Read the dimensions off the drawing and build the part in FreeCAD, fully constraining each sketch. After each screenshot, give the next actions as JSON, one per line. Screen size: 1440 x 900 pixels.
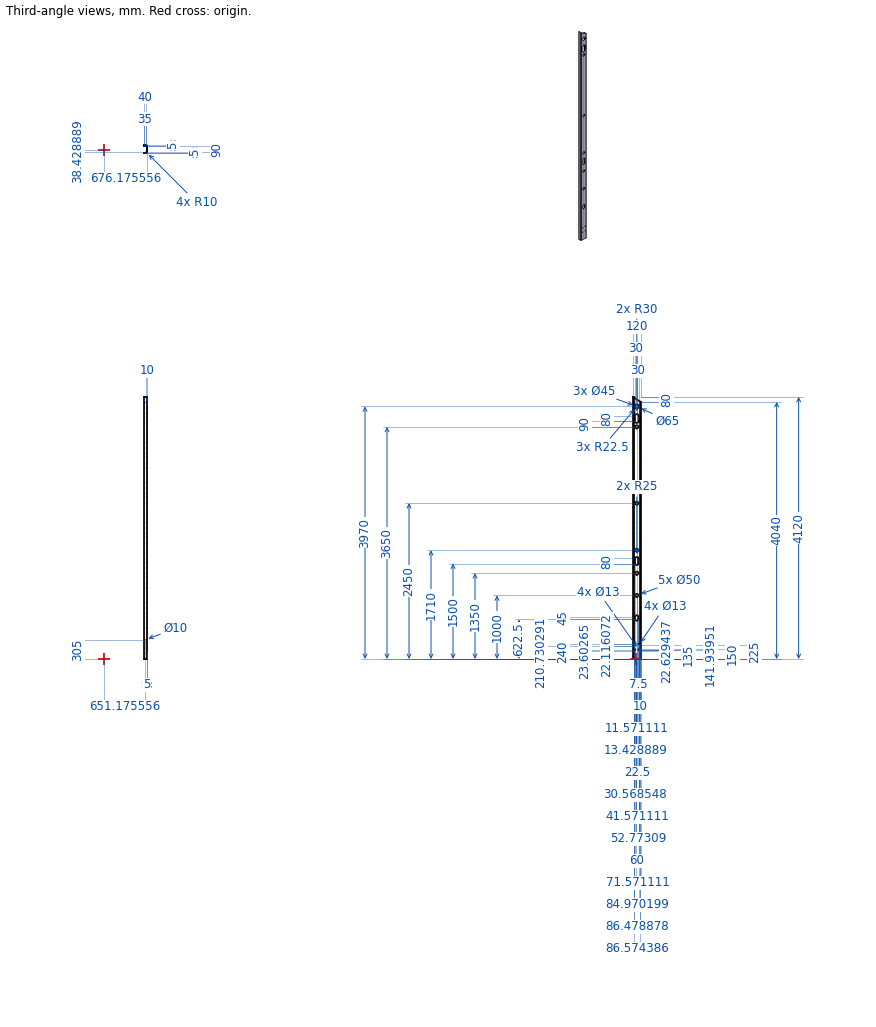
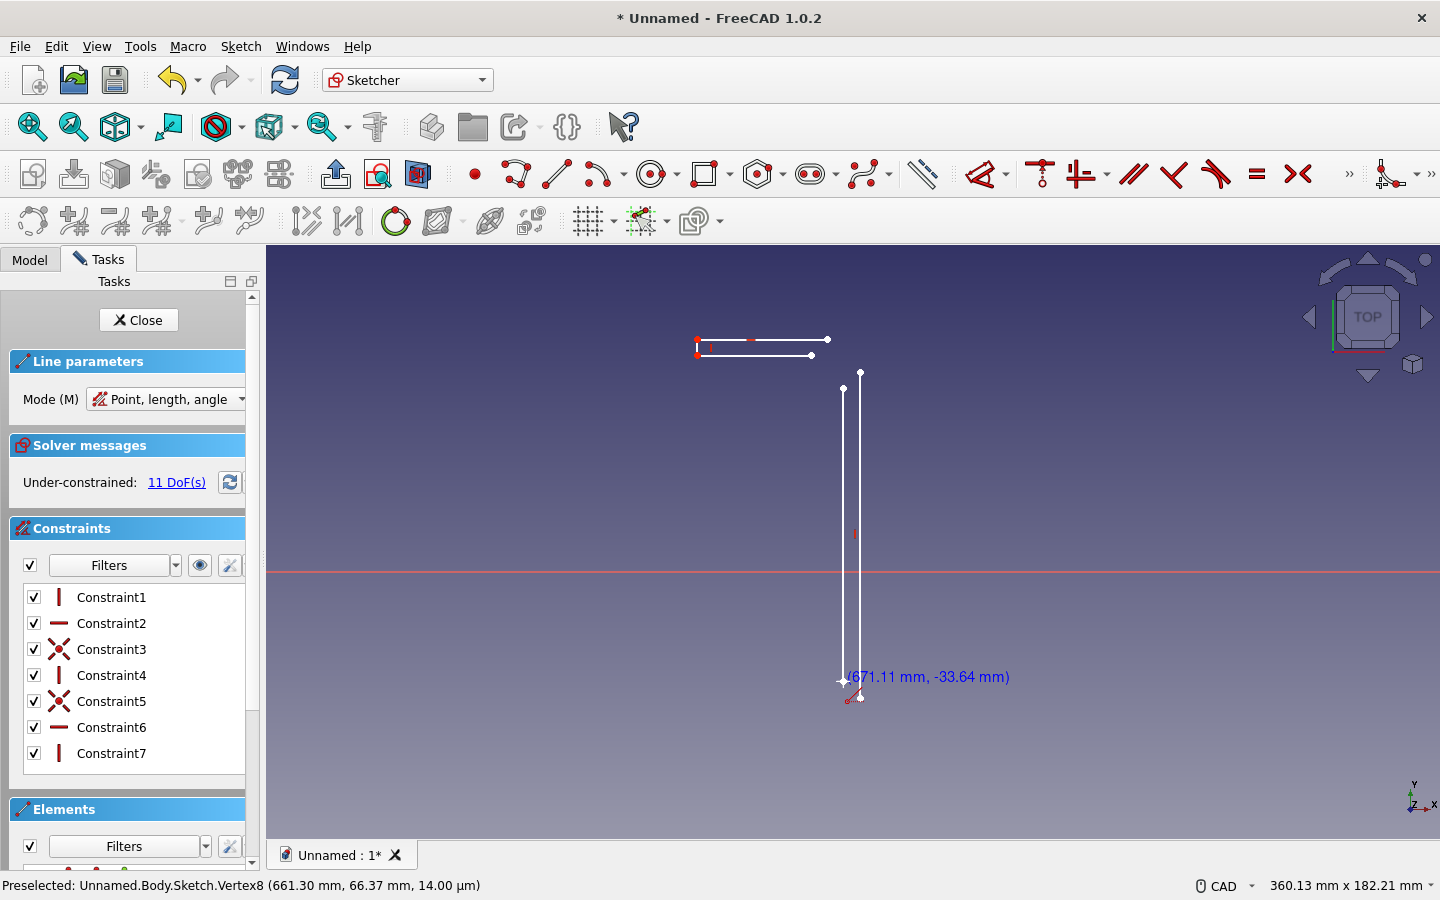
{"action": "key", "text": "g m"}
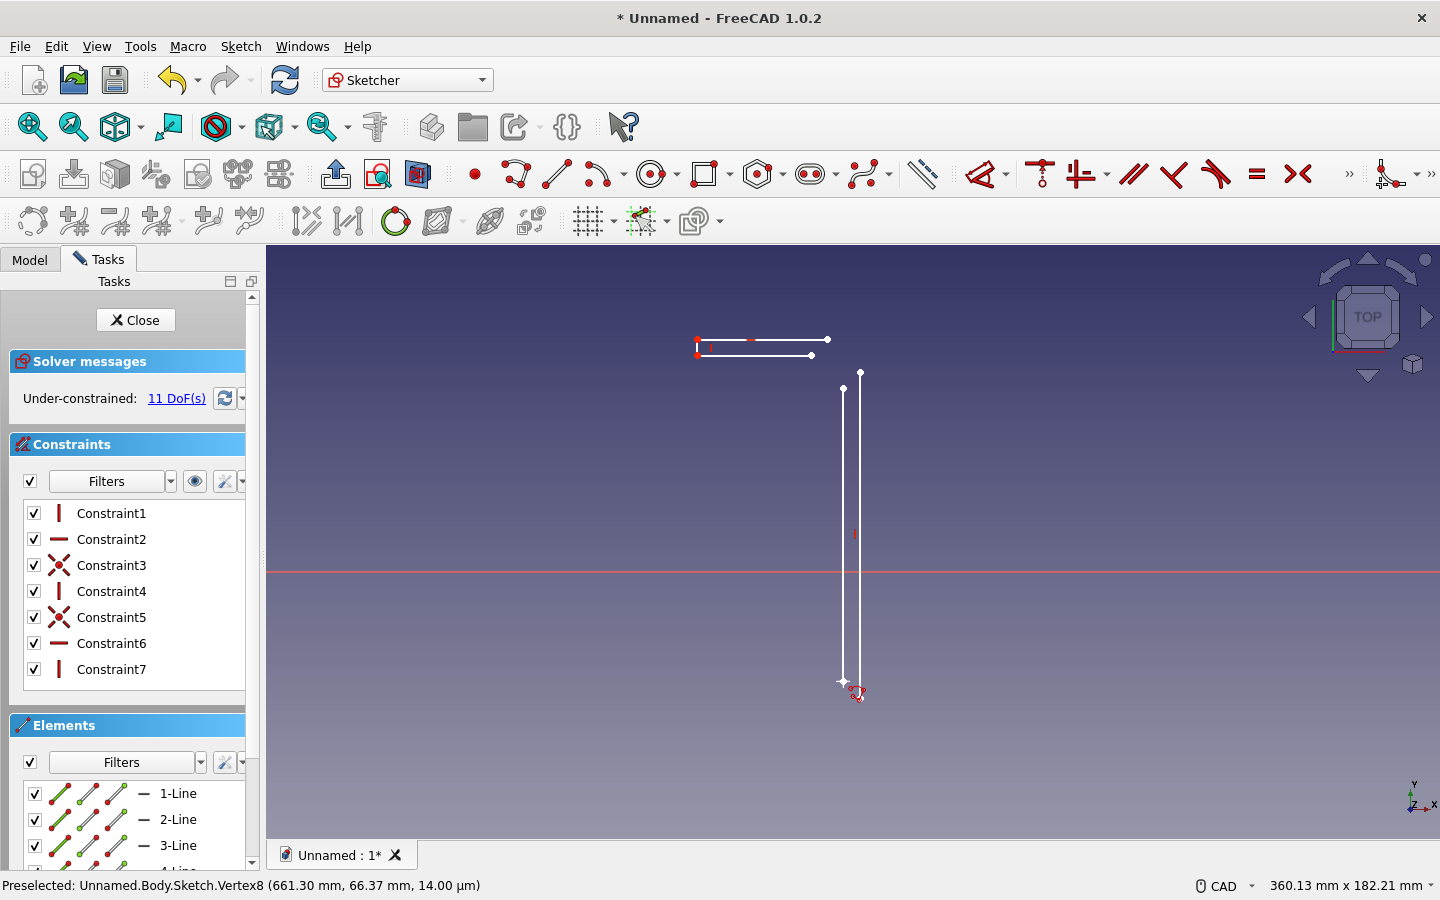
{"action": "left_click", "coordinate": [811, 714]}
{"action": "left_click", "coordinate": [697, 714]}
{"action": "left_click", "coordinate": [697, 730]}
{"action": "left_click", "coordinate": [827, 730]}
{"action": "right_click", "coordinate": [827, 730]}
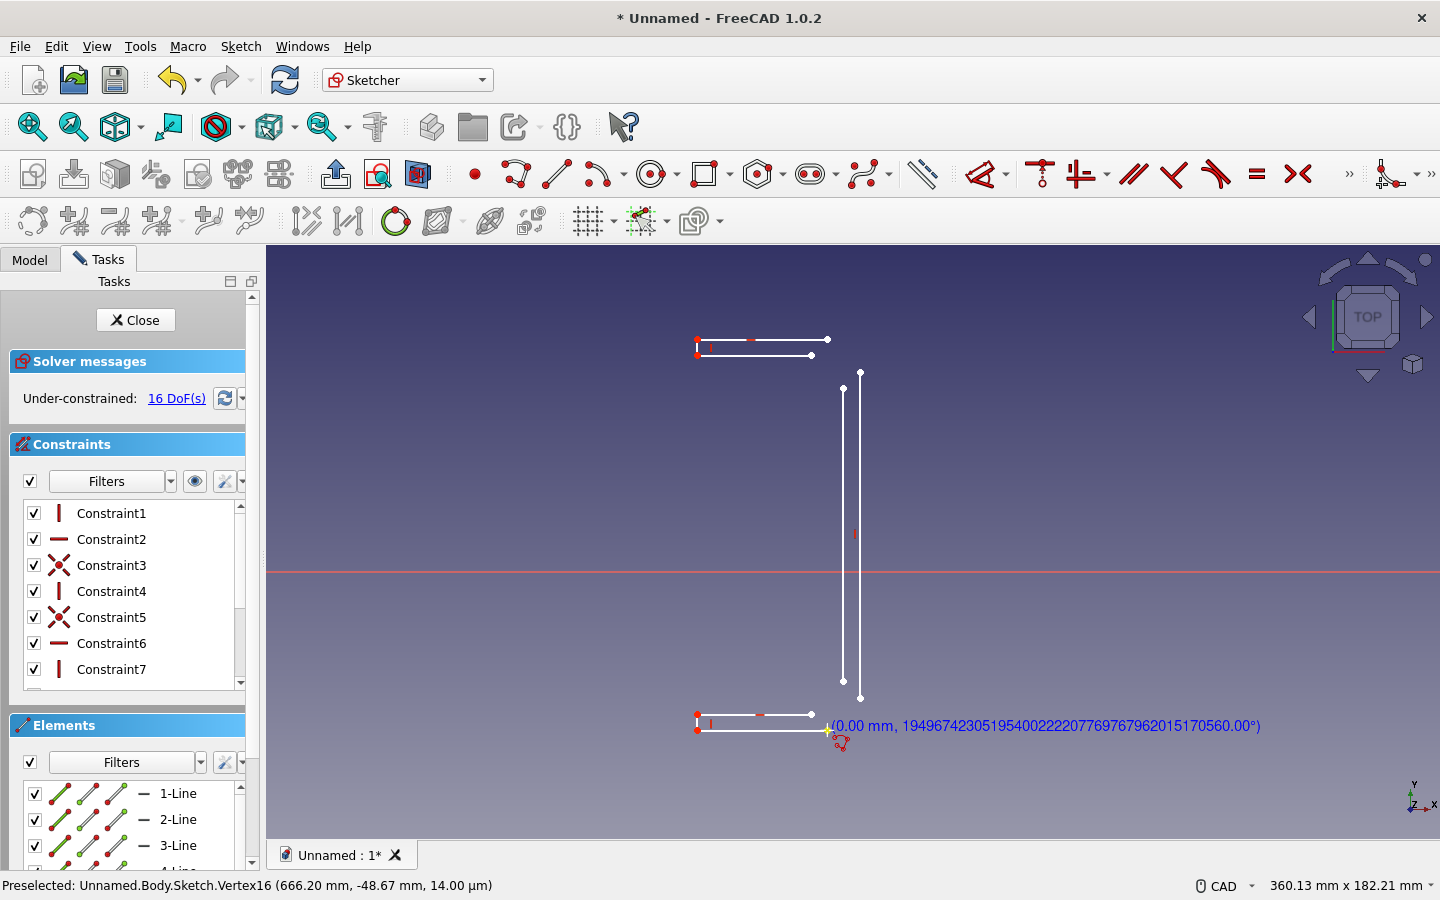
{"action": "key", "text": "g 3 a"}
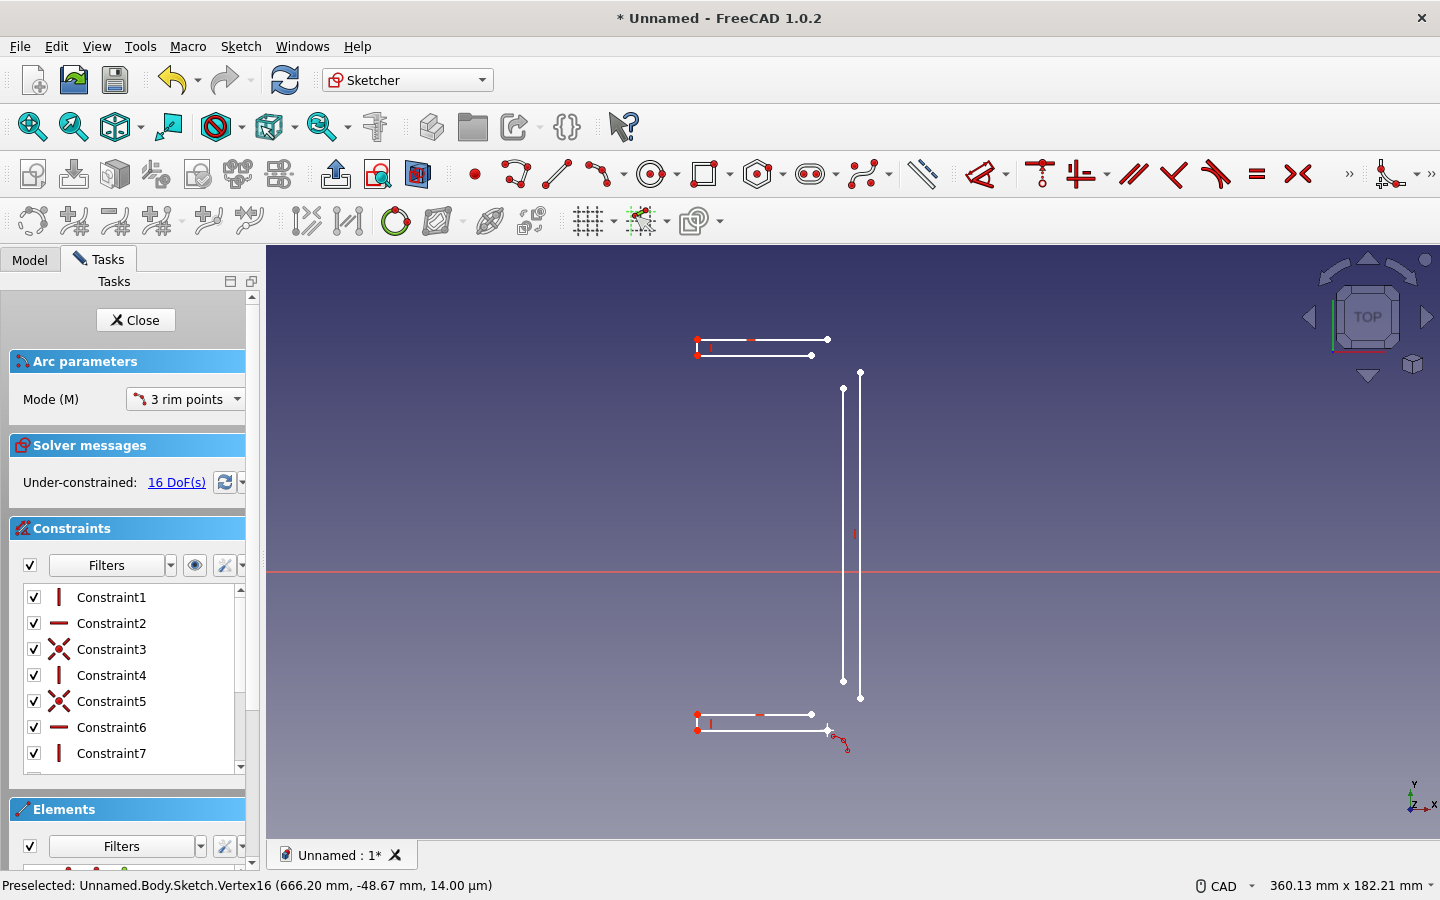
{"action": "left_click", "coordinate": [860, 373]}
{"action": "left_click", "coordinate": [827, 340]}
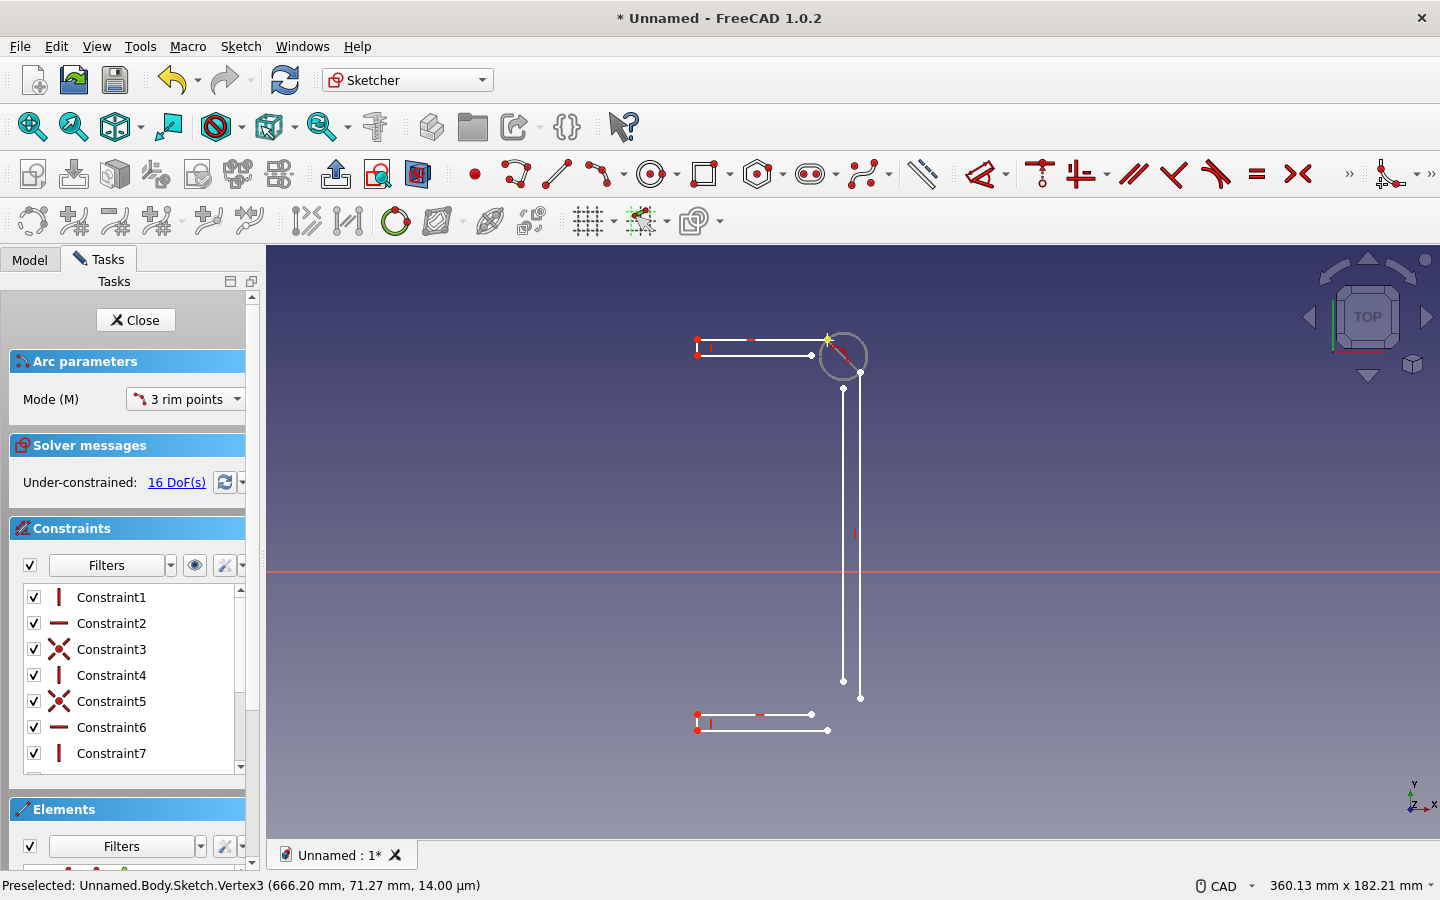
{"action": "scroll", "coordinate": [850, 349], "scroll_direction": "up", "scroll_amount": 3}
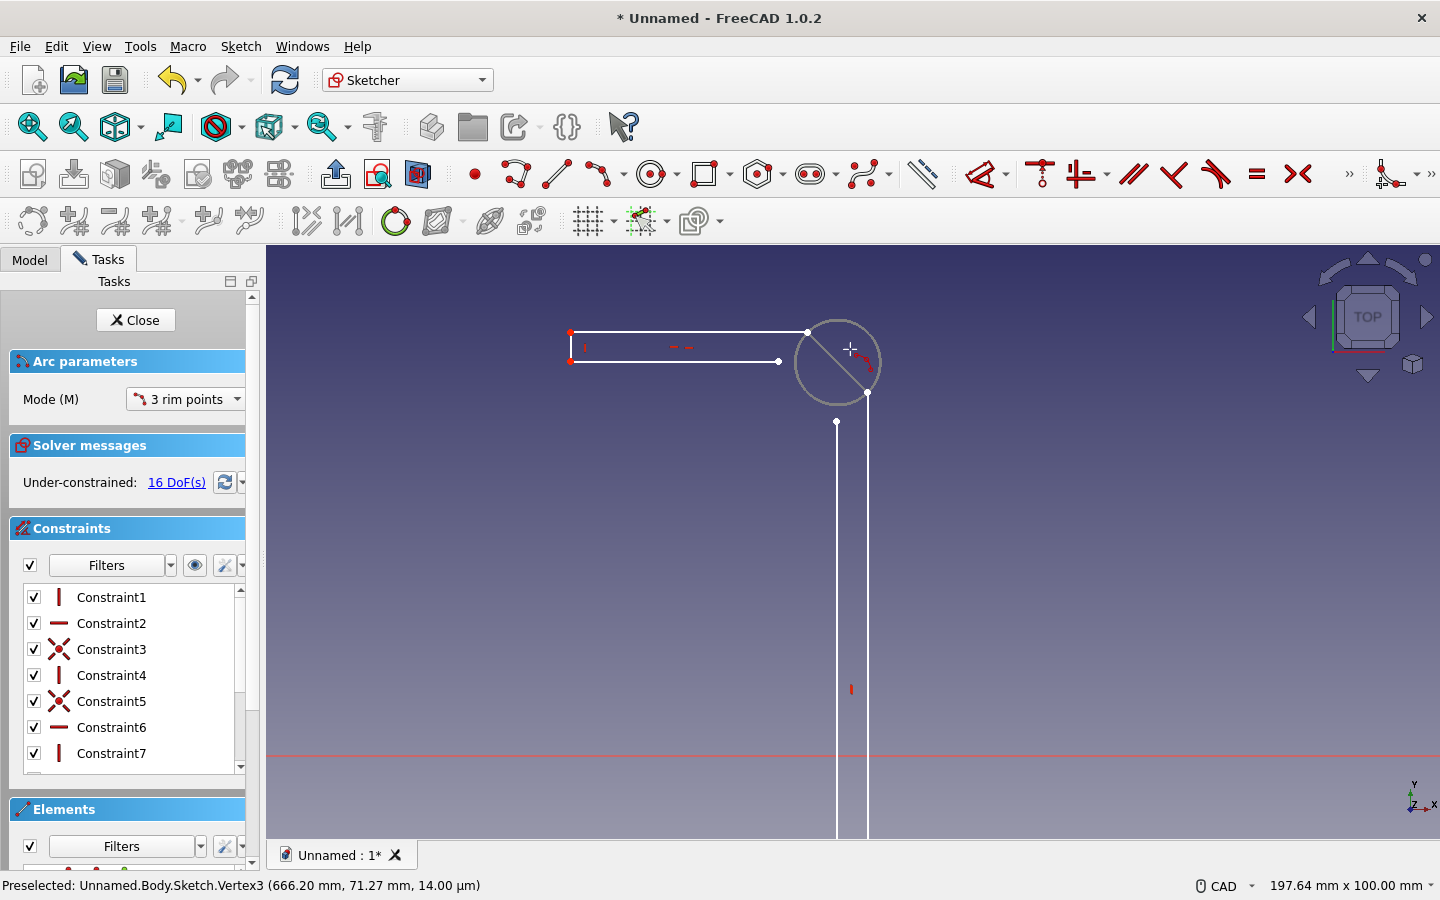
{"action": "left_click", "coordinate": [850, 348]}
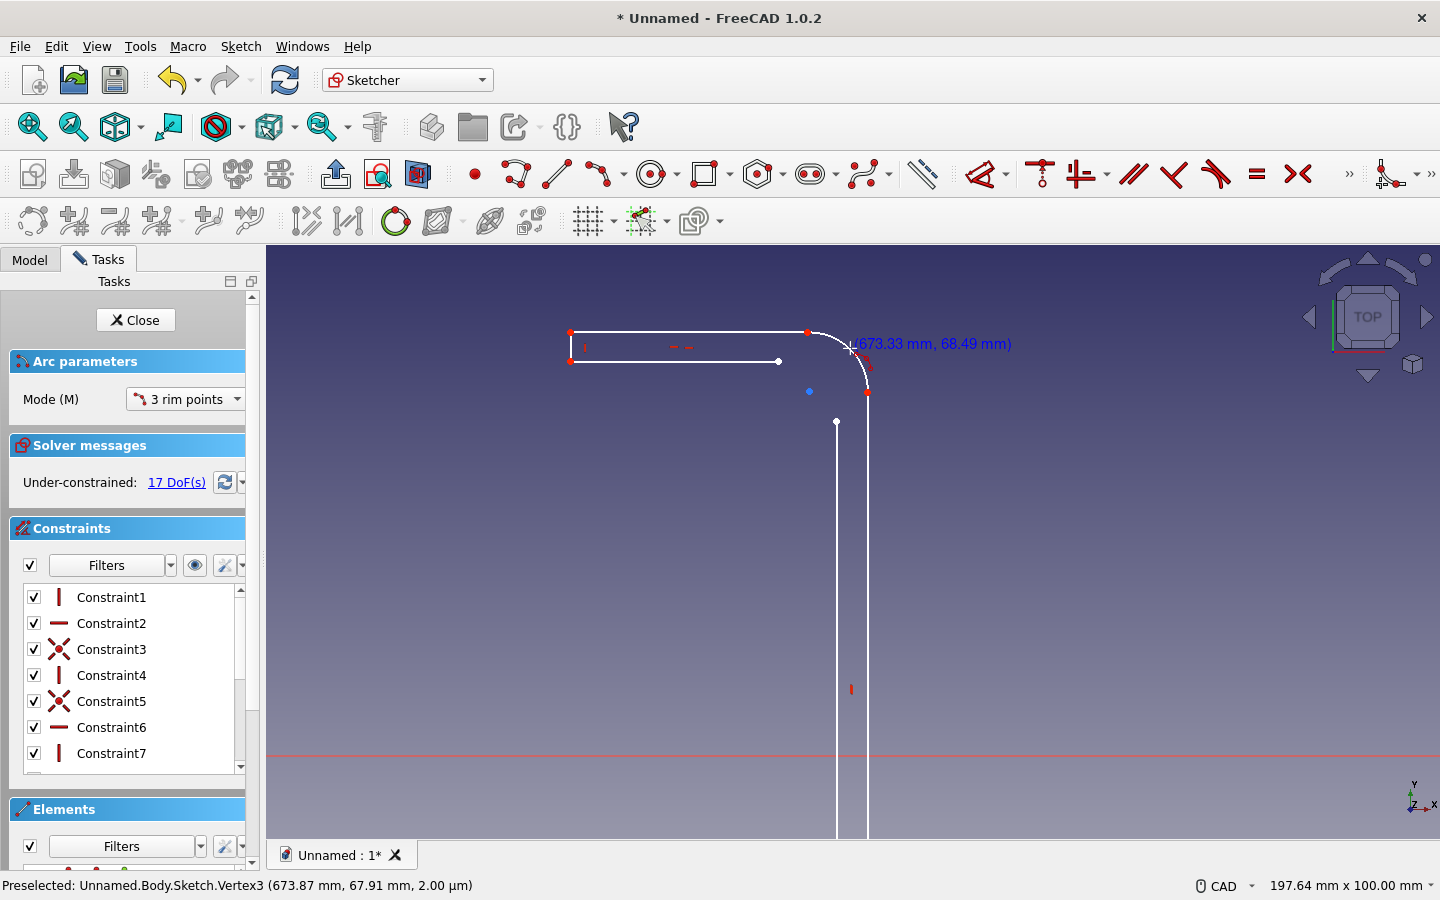
{"action": "left_click", "coordinate": [779, 362]}
{"action": "left_click", "coordinate": [837, 422]}
{"action": "left_click", "coordinate": [820, 378]}